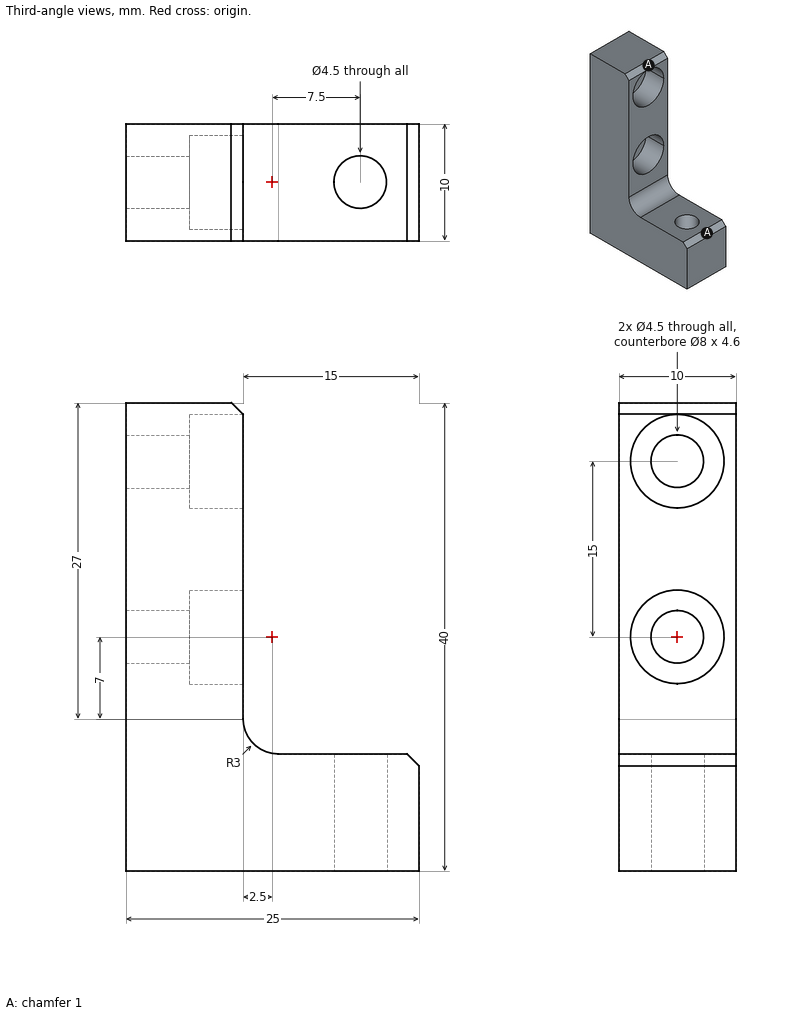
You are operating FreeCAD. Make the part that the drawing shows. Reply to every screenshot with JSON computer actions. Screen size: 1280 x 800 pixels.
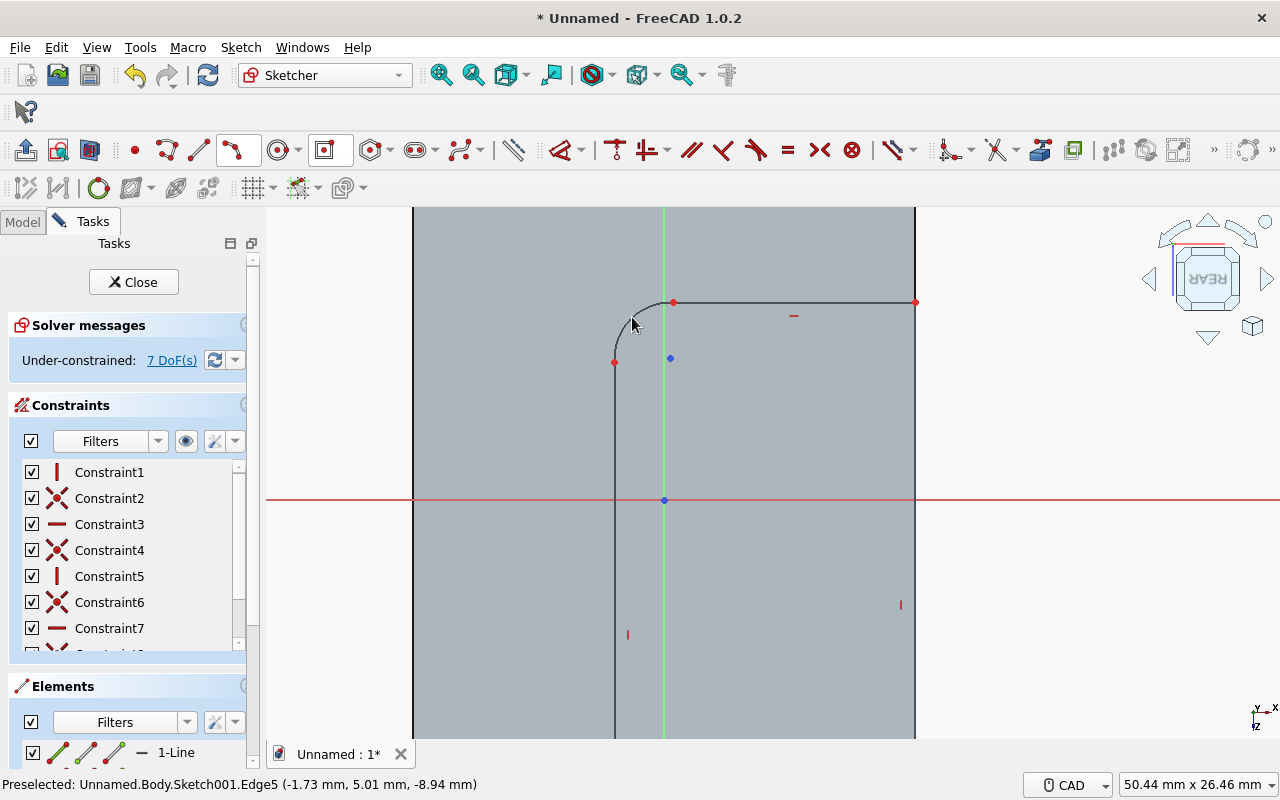
{"action": "left_click", "coordinate": [615, 526]}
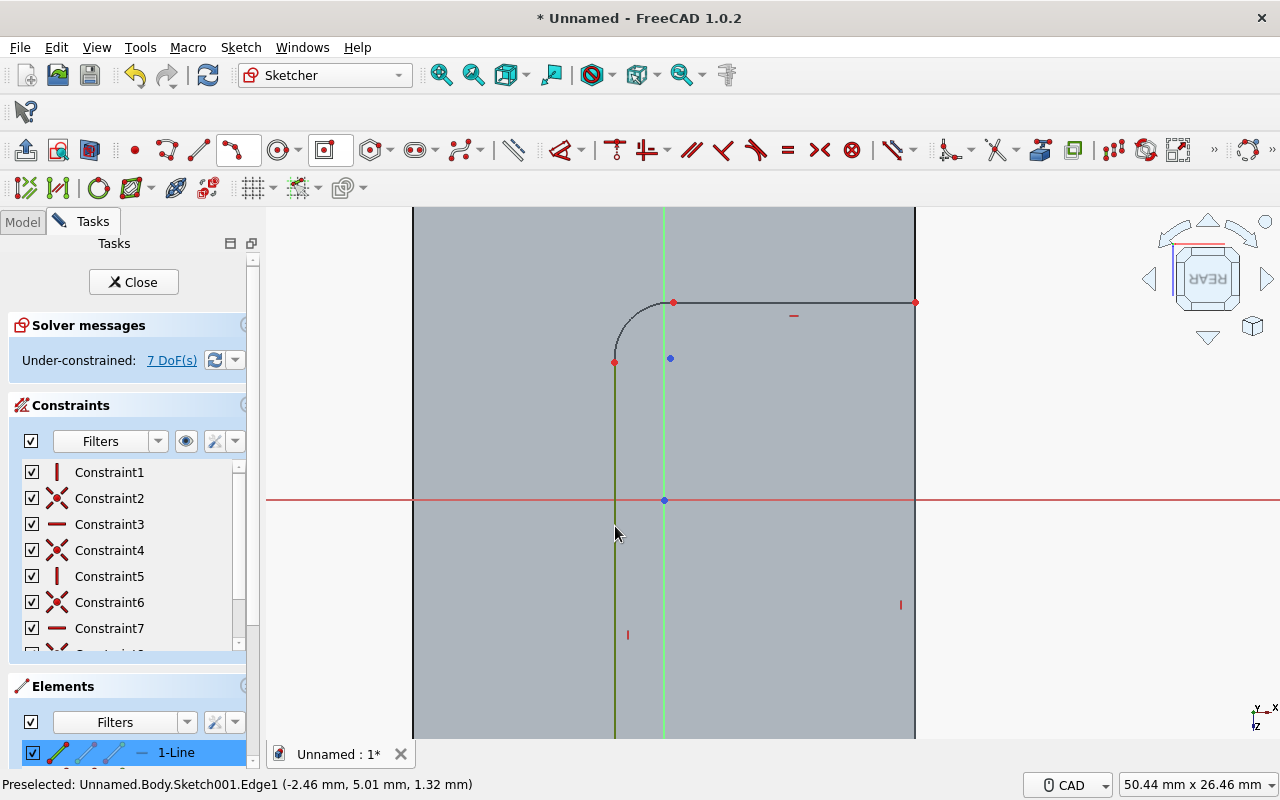
{"action": "left_click", "coordinate": [646, 308]}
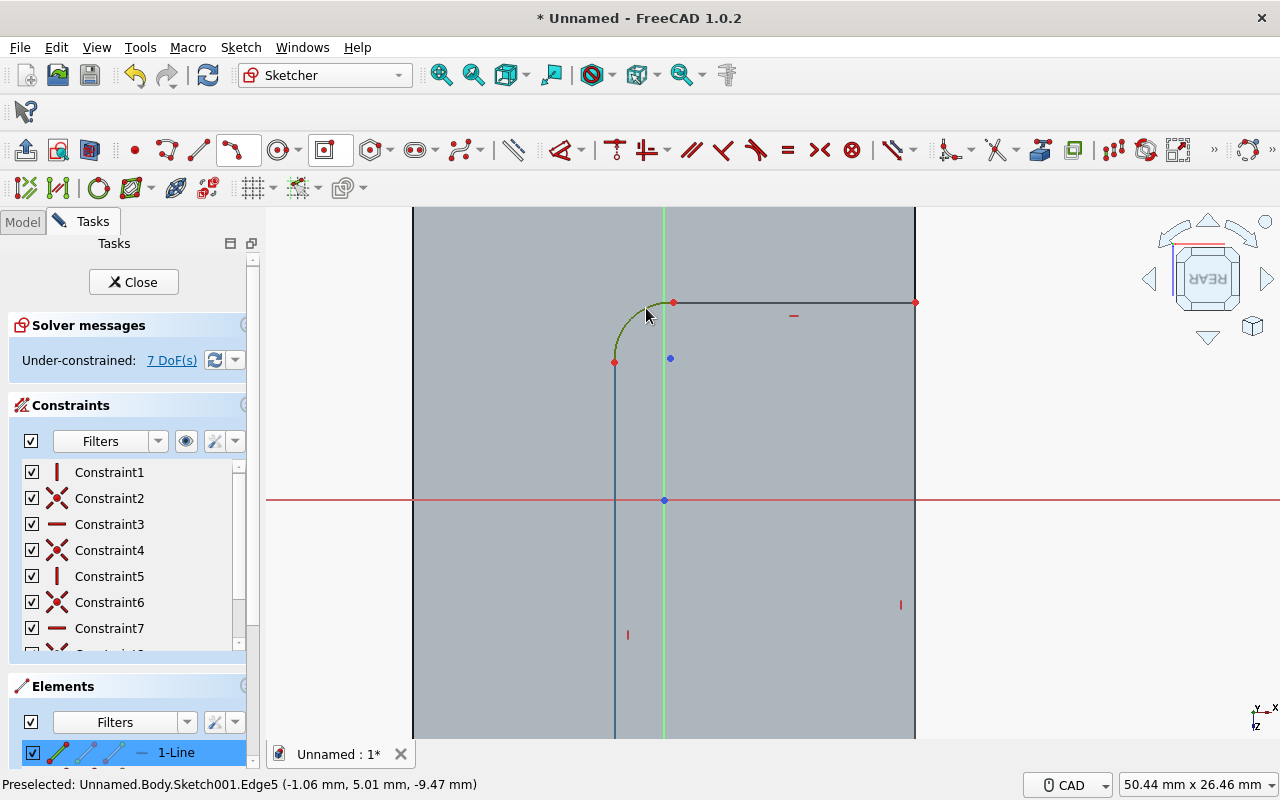
{"action": "left_click", "coordinate": [756, 150]}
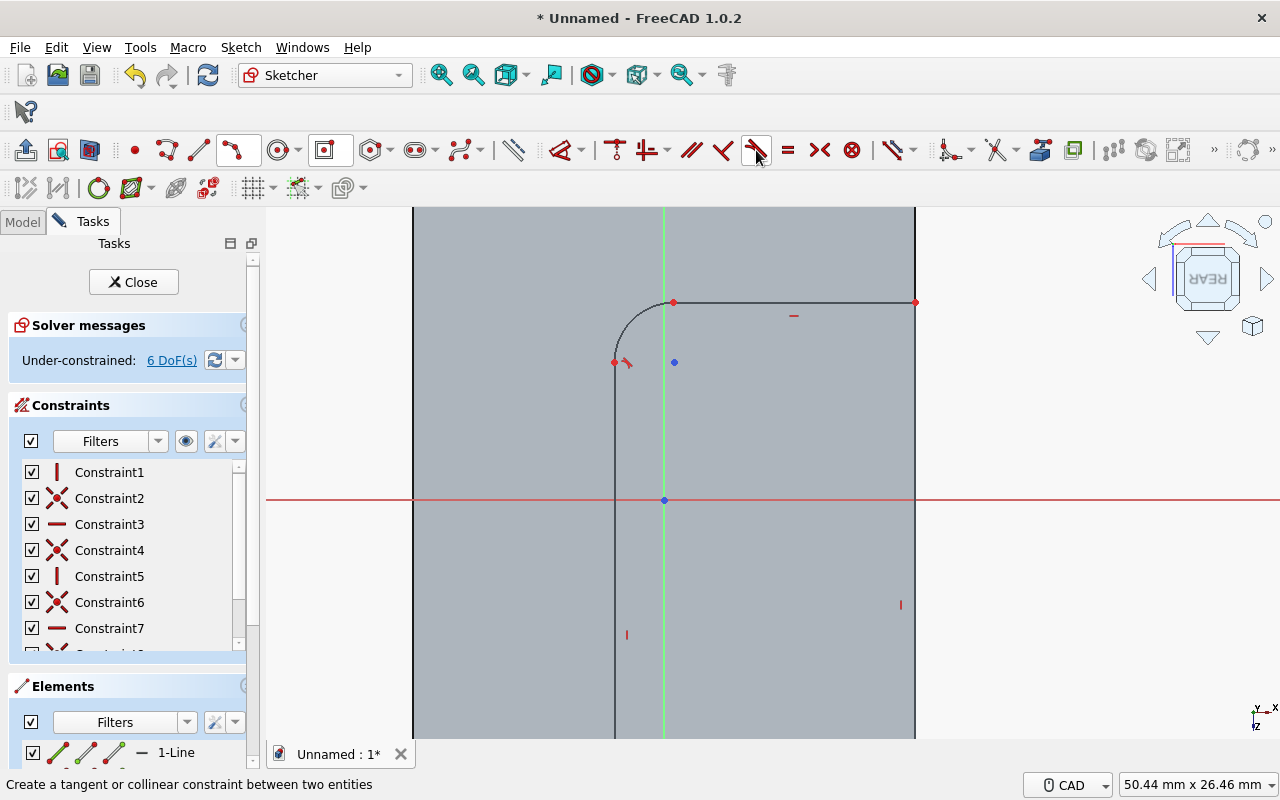
{"action": "left_click", "coordinate": [843, 303]}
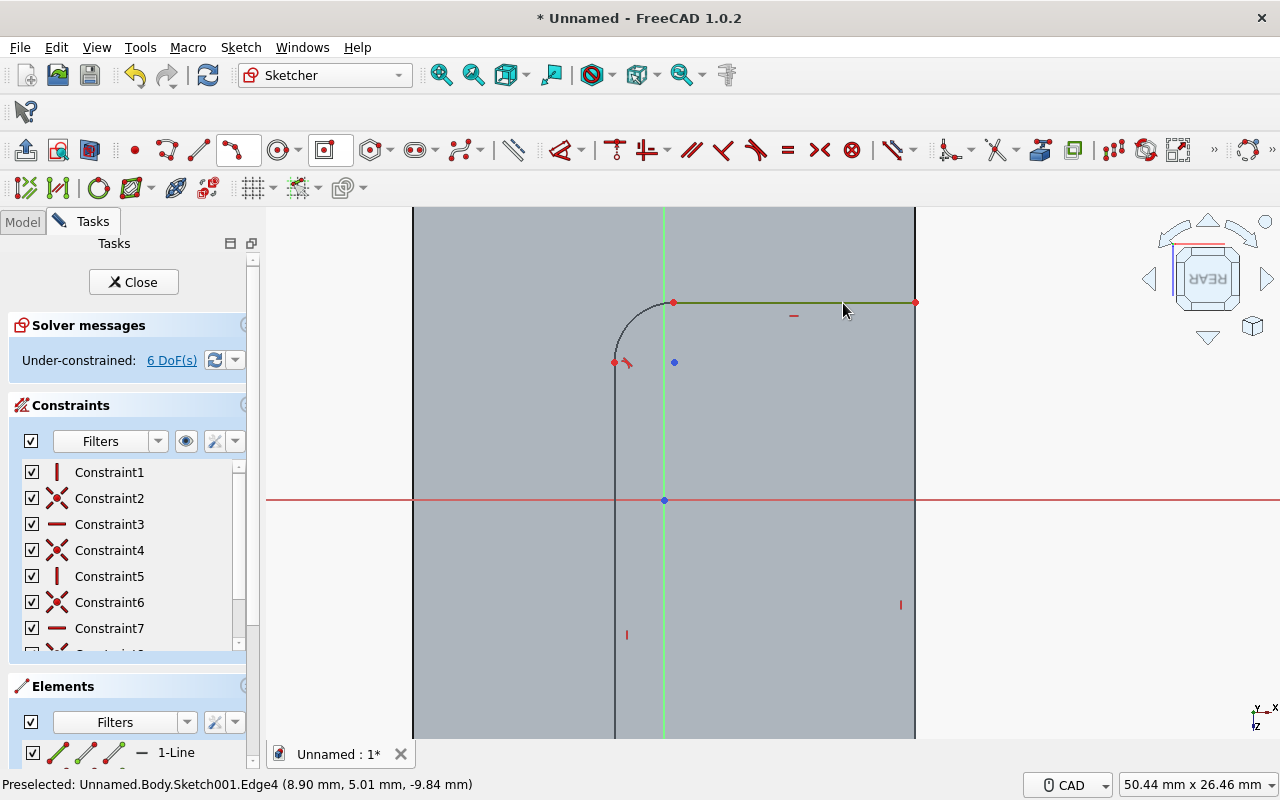
{"action": "left_click", "coordinate": [647, 309]}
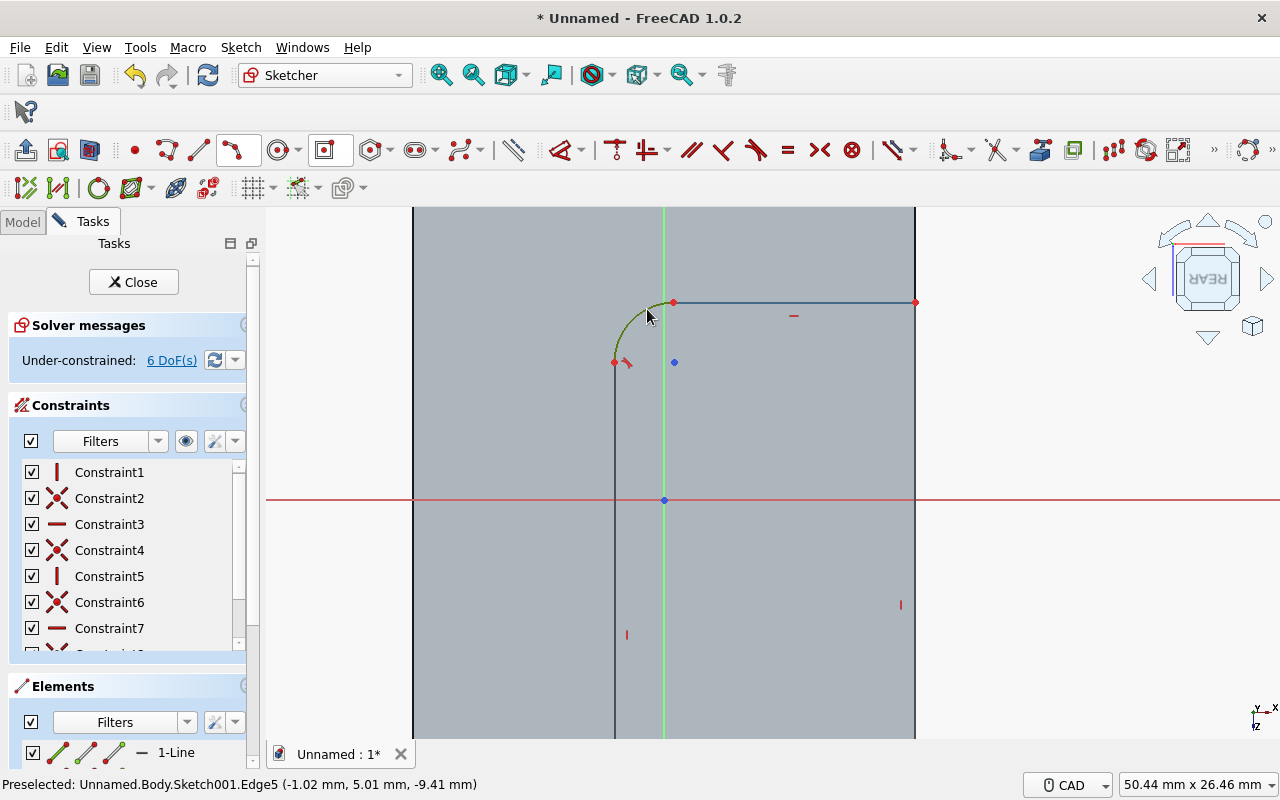
{"action": "left_click", "coordinate": [756, 150]}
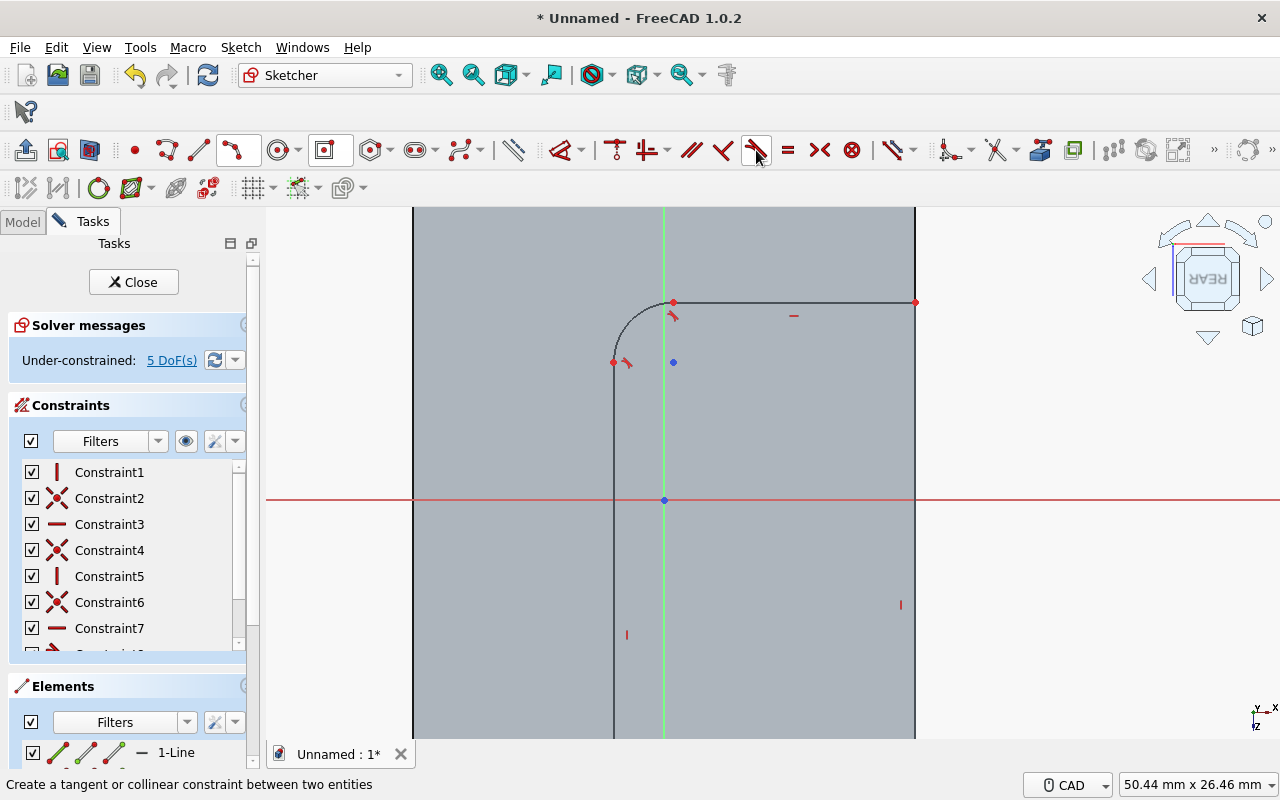
{"action": "key", "text": "d"}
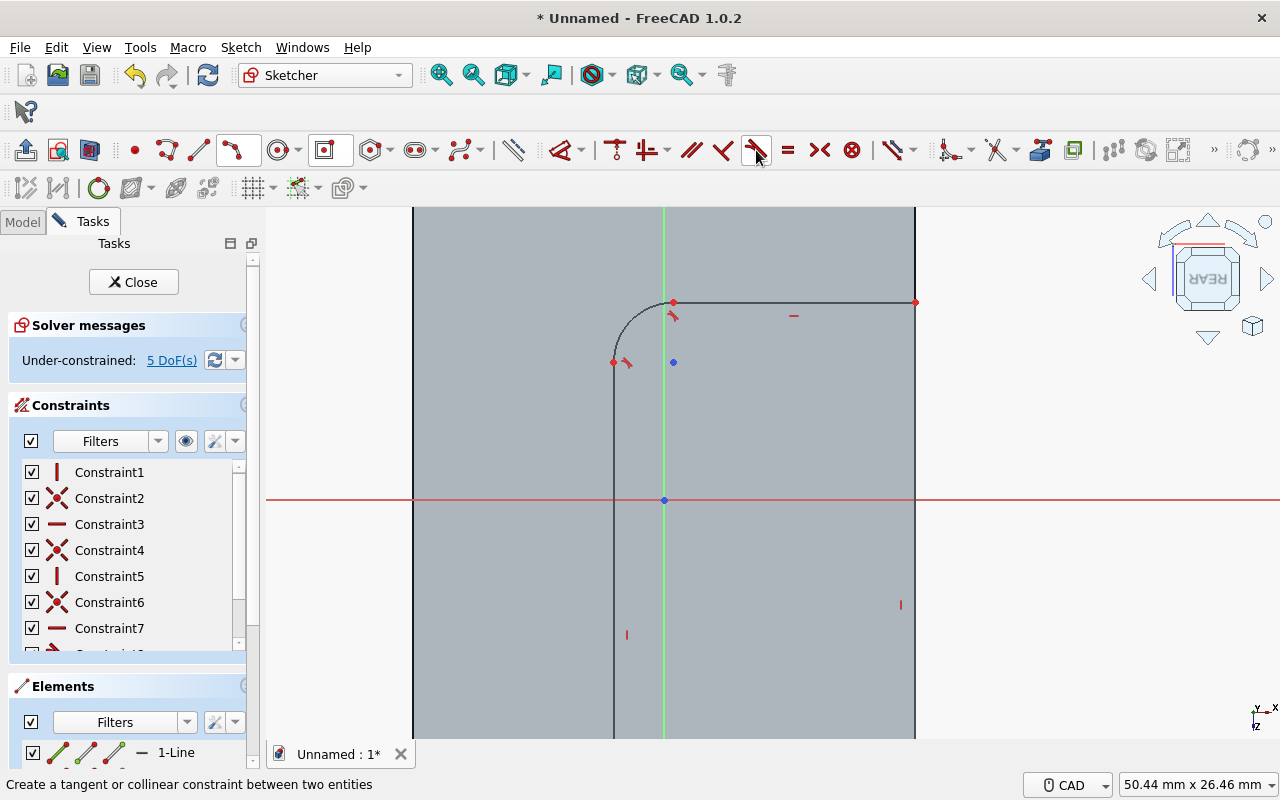
{"action": "left_click", "coordinate": [647, 309]}
{"action": "left_click", "coordinate": [633, 280]}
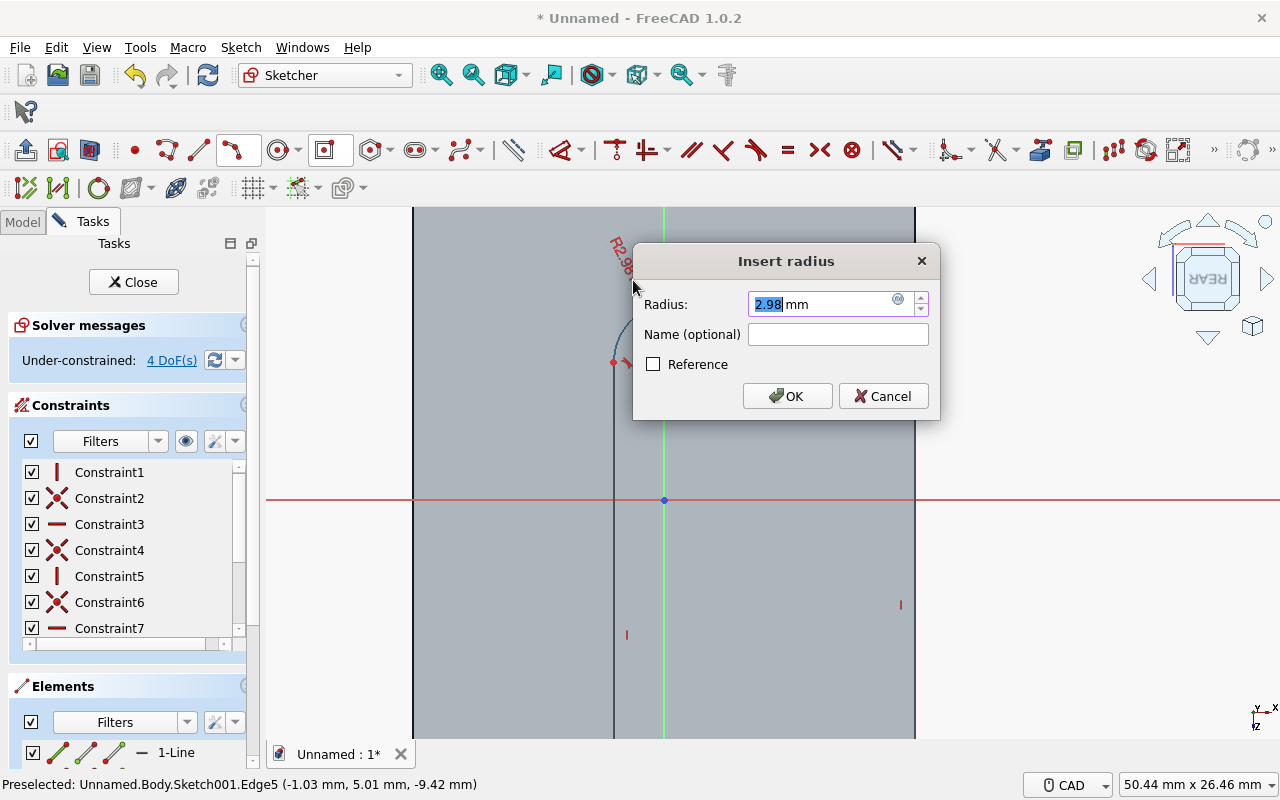
{"action": "type", "text": "3"}
{"action": "key", "text": "Return"}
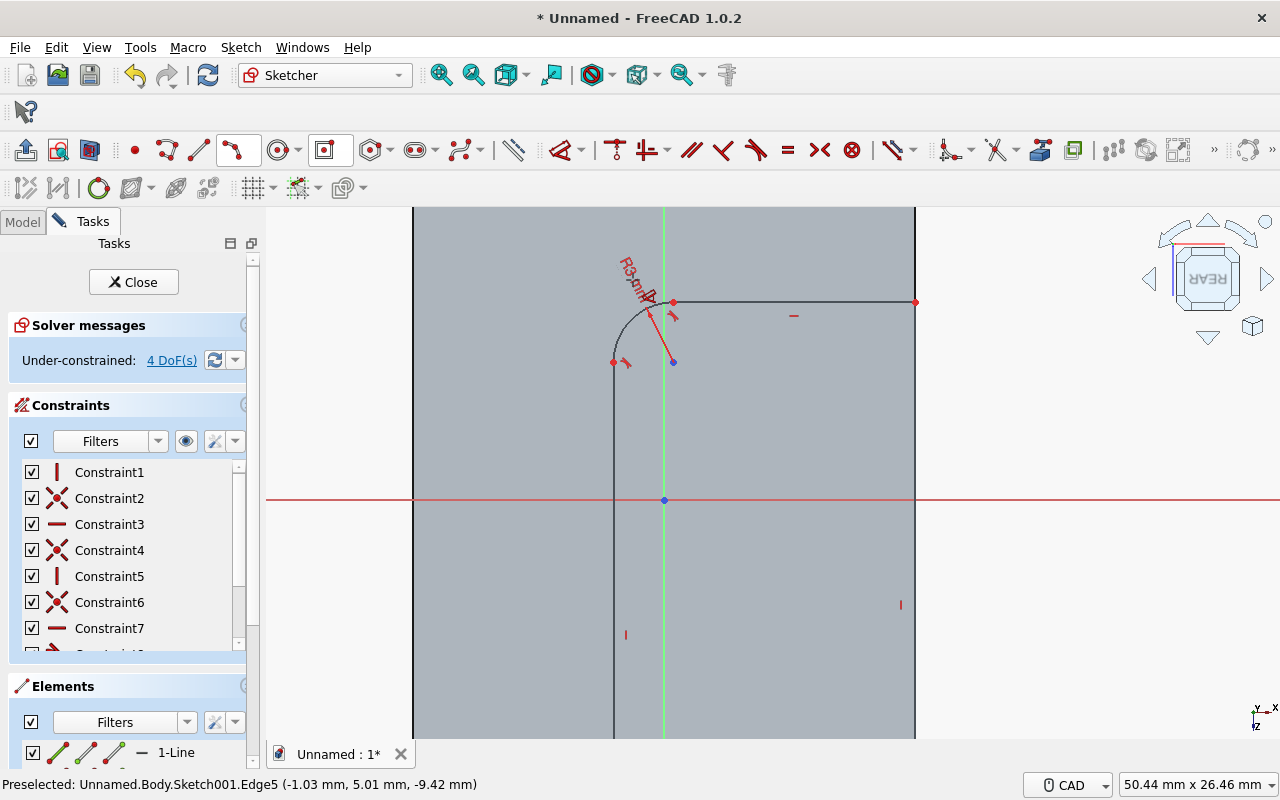
{"action": "left_click", "coordinate": [614, 526]}
{"action": "left_click", "coordinate": [580, 537]}